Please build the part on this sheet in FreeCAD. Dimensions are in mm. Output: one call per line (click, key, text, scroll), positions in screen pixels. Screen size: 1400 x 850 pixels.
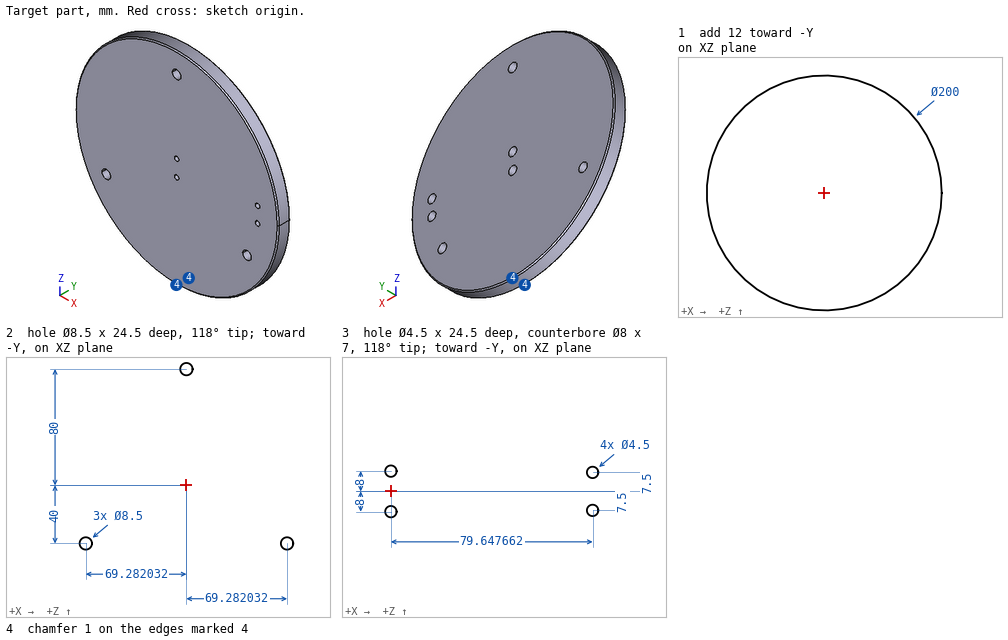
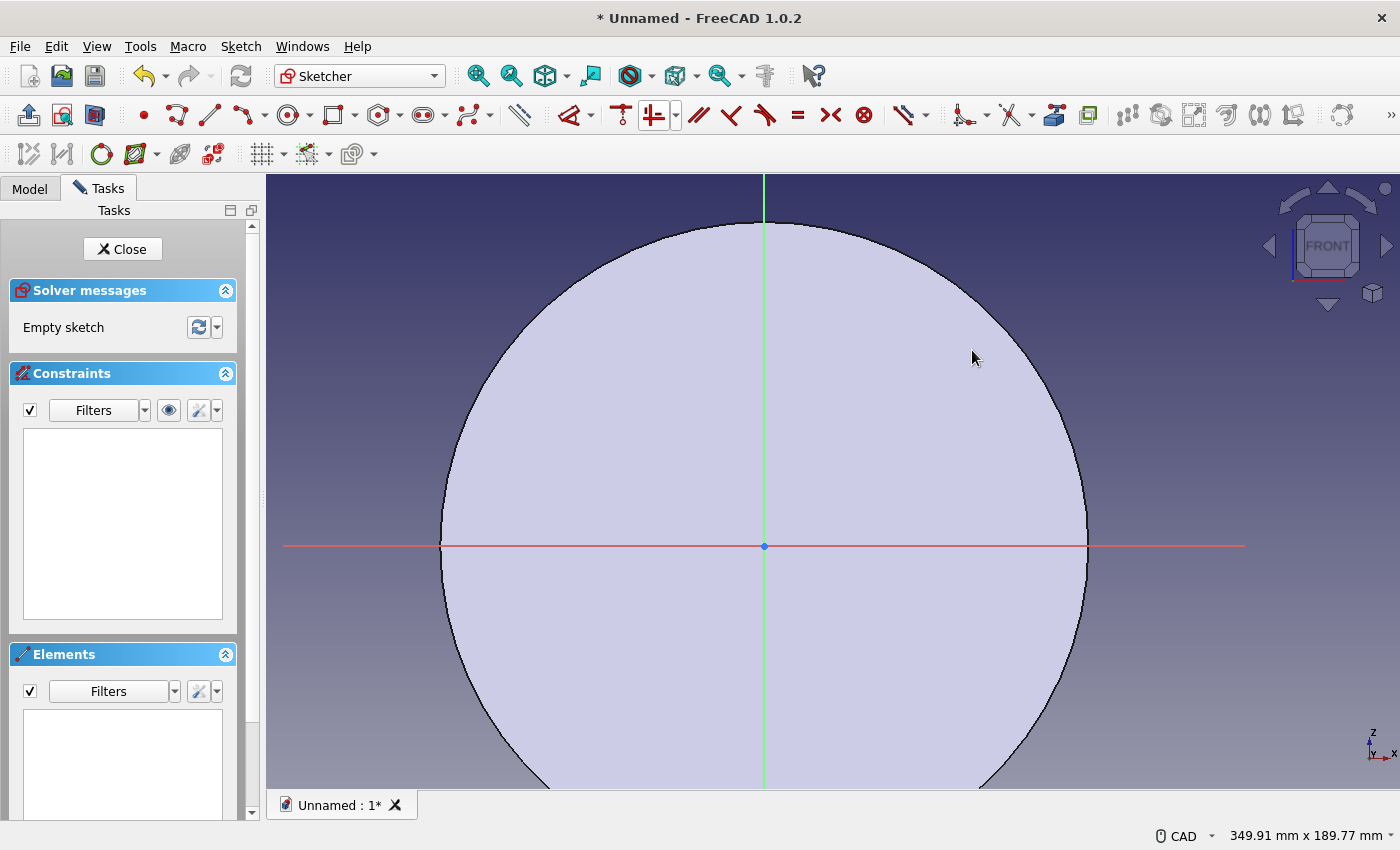
click(288, 116)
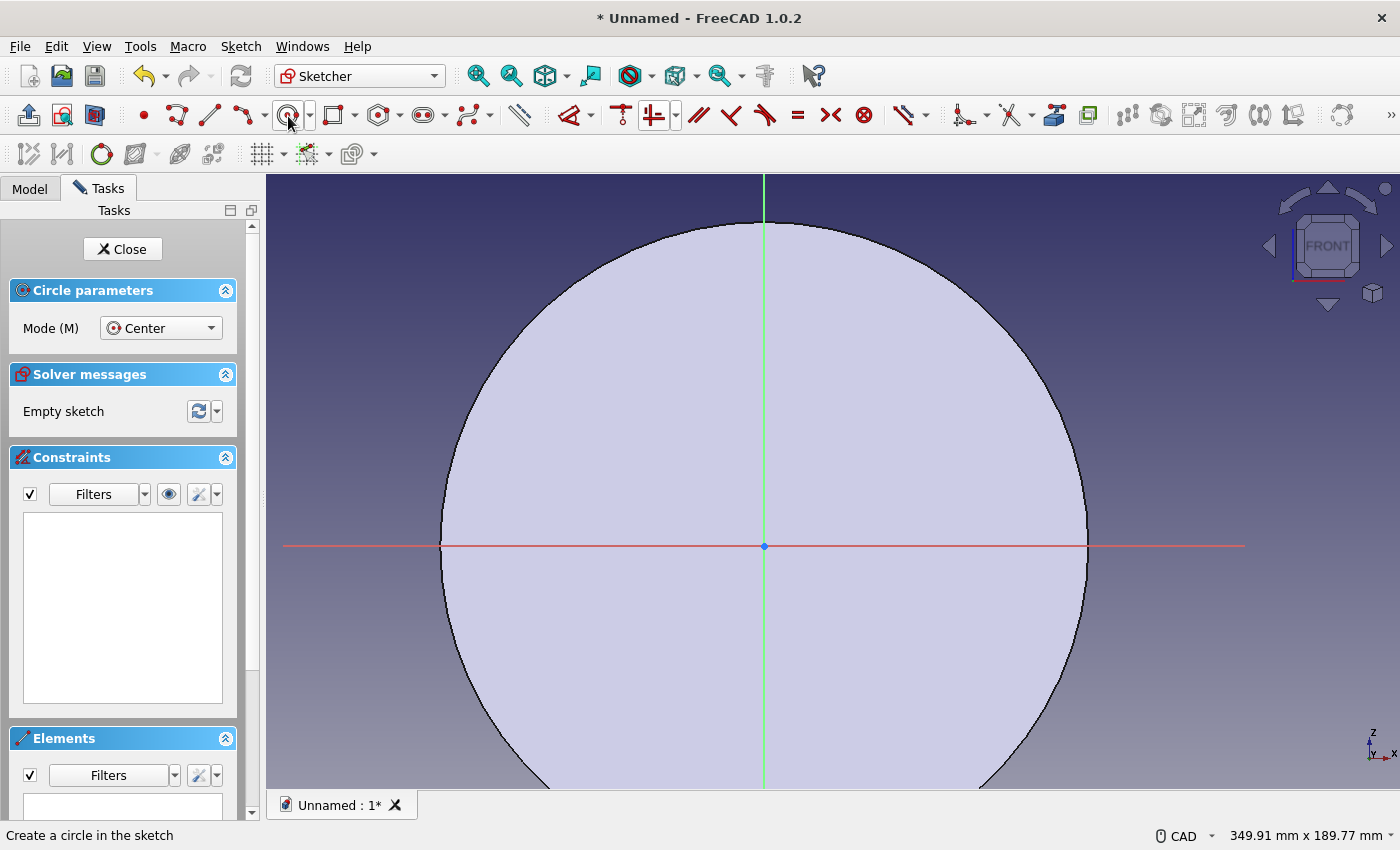
scroll(540, 676, up, 3)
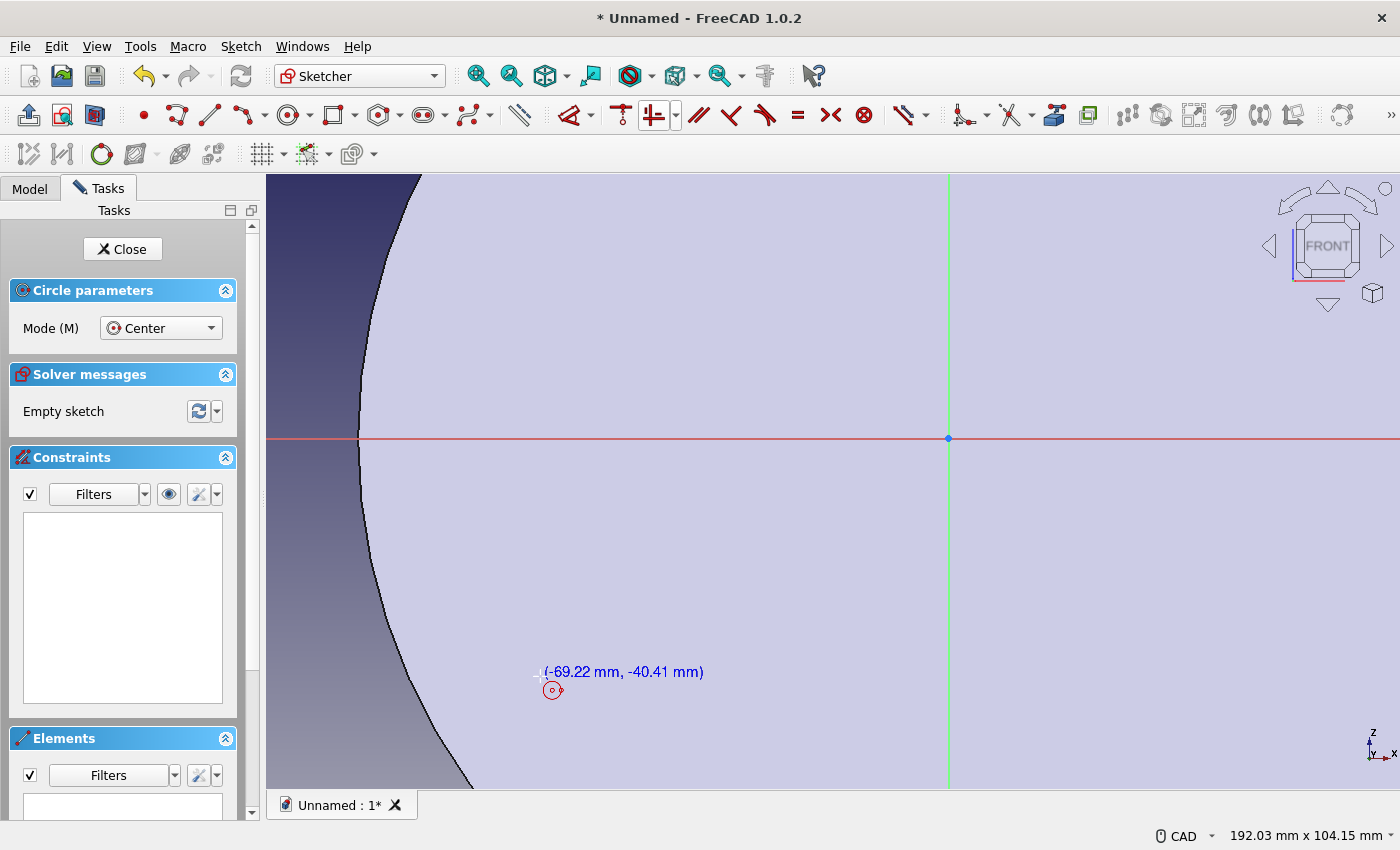
click(539, 675)
move(557, 657)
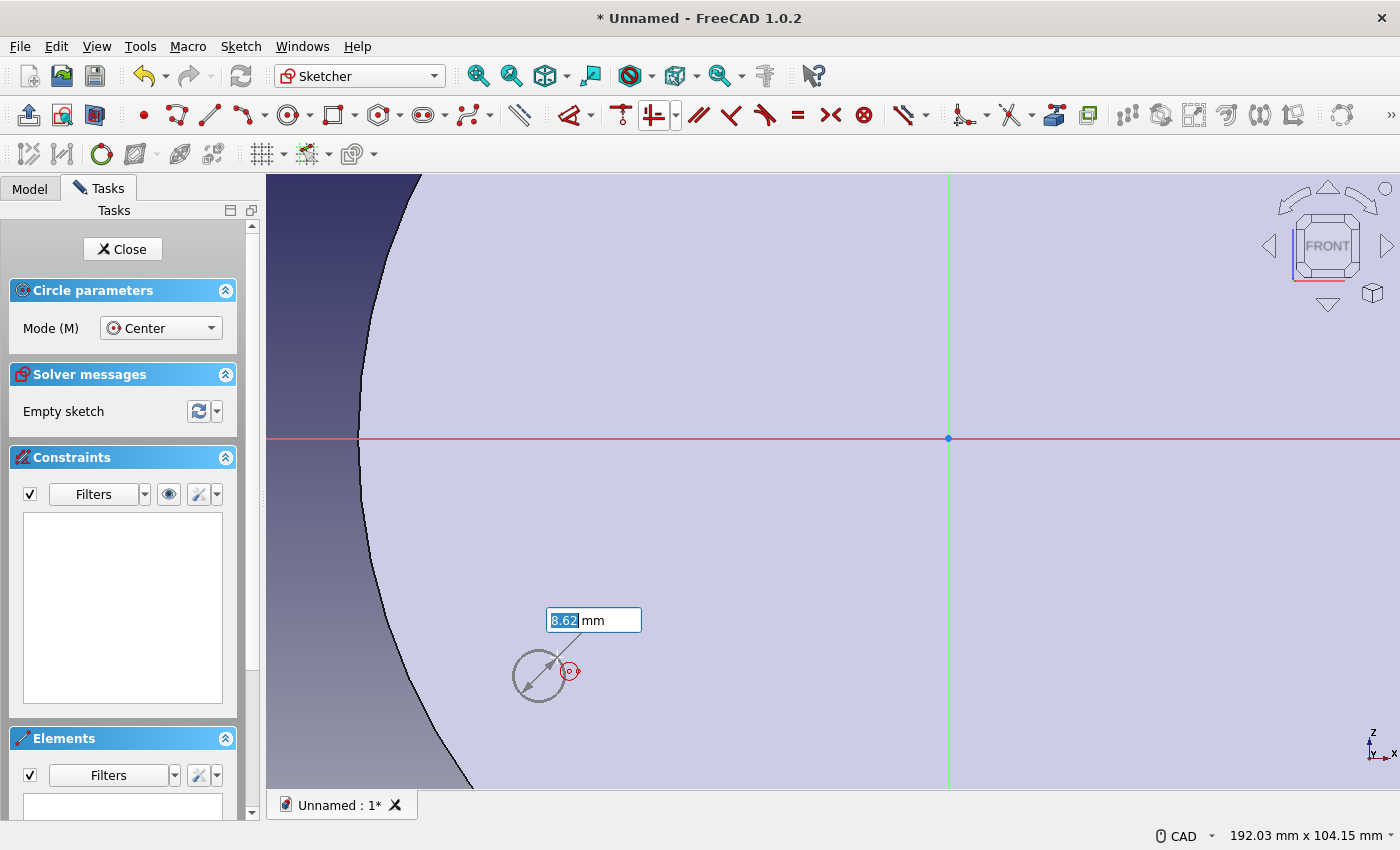
text(8.5)
key(Return)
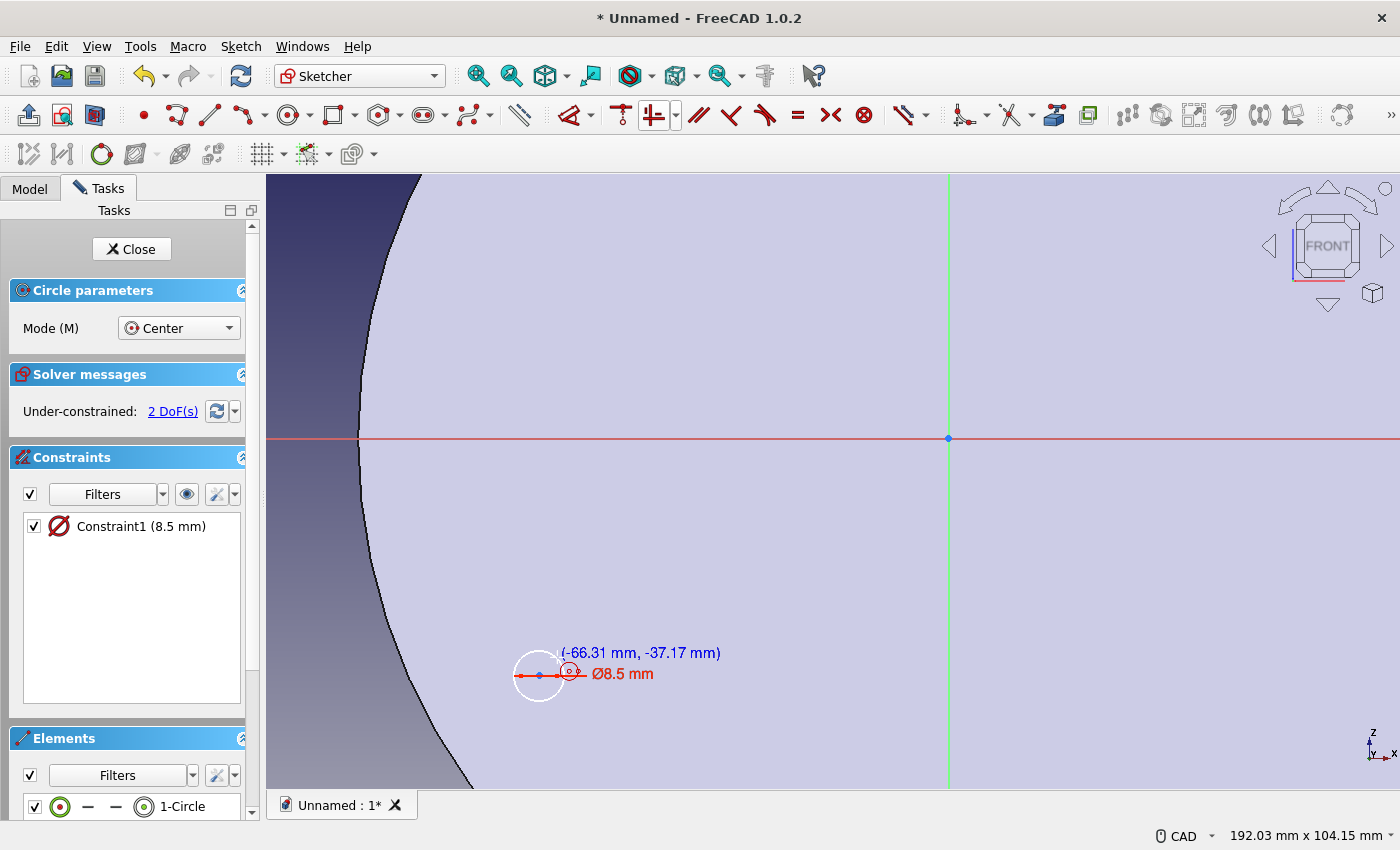
scroll(541, 677, down, 3)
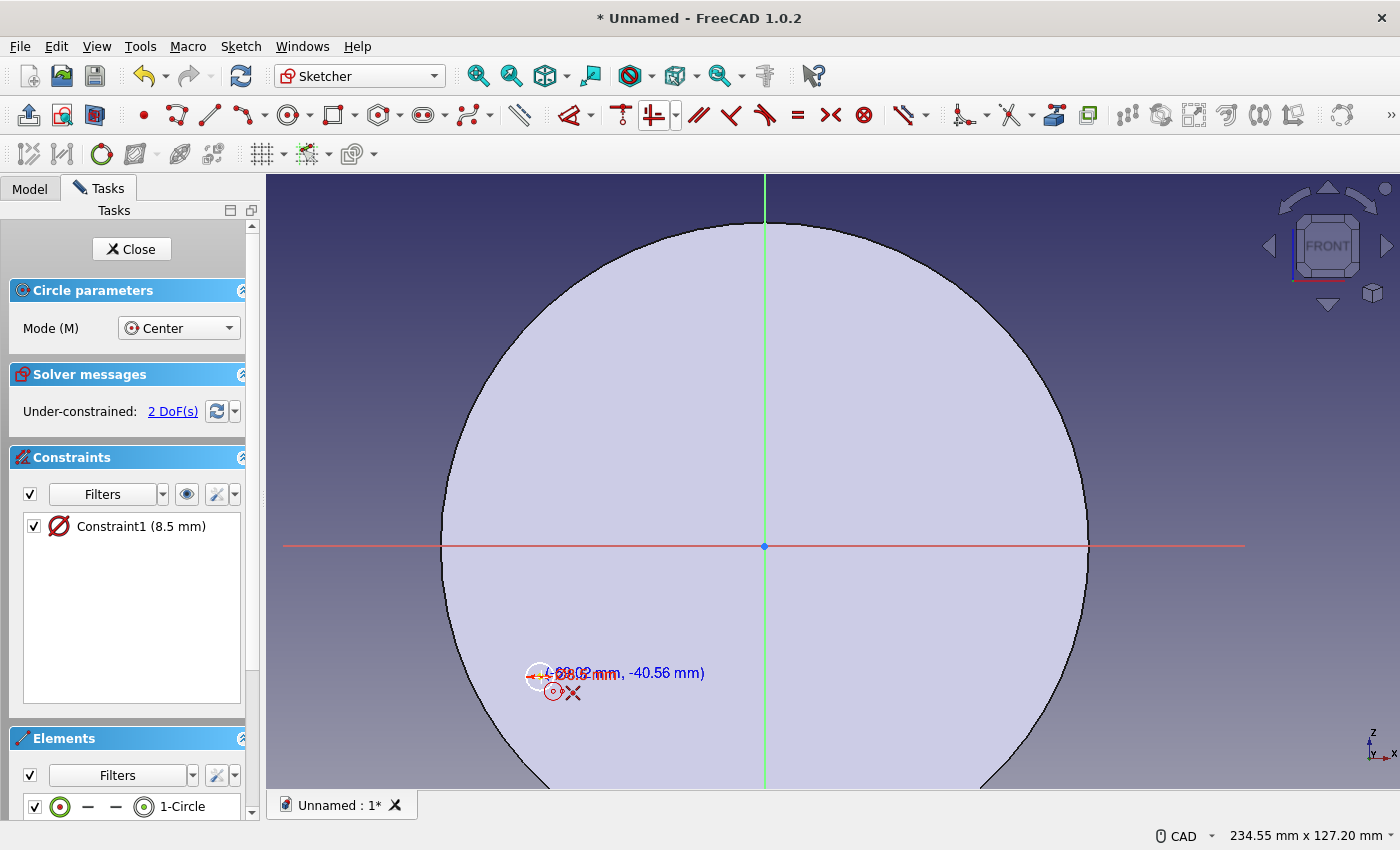
scroll(989, 676, up, 3)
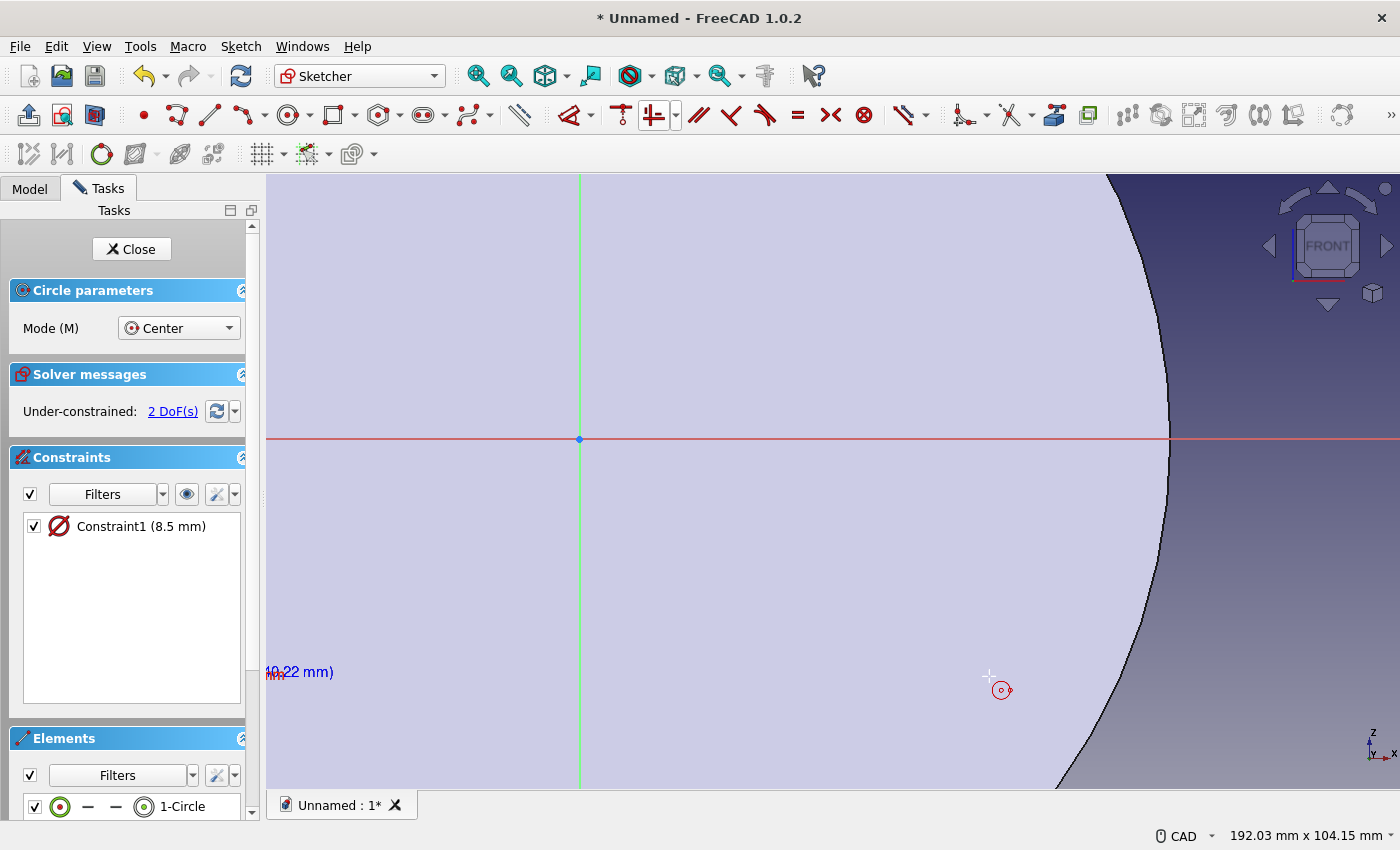
click(989, 676)
move(1007, 658)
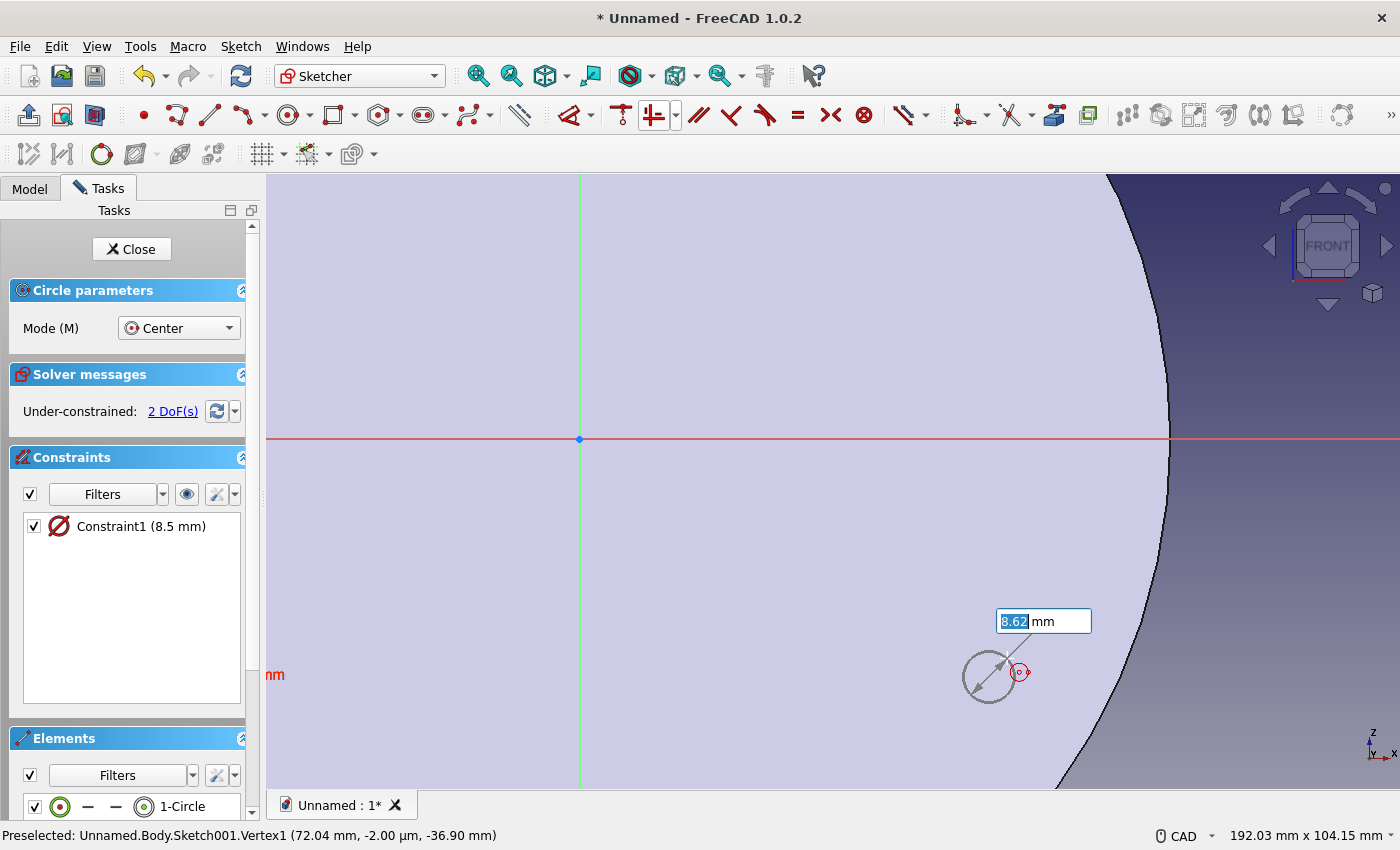
text(8.5)
key(Return)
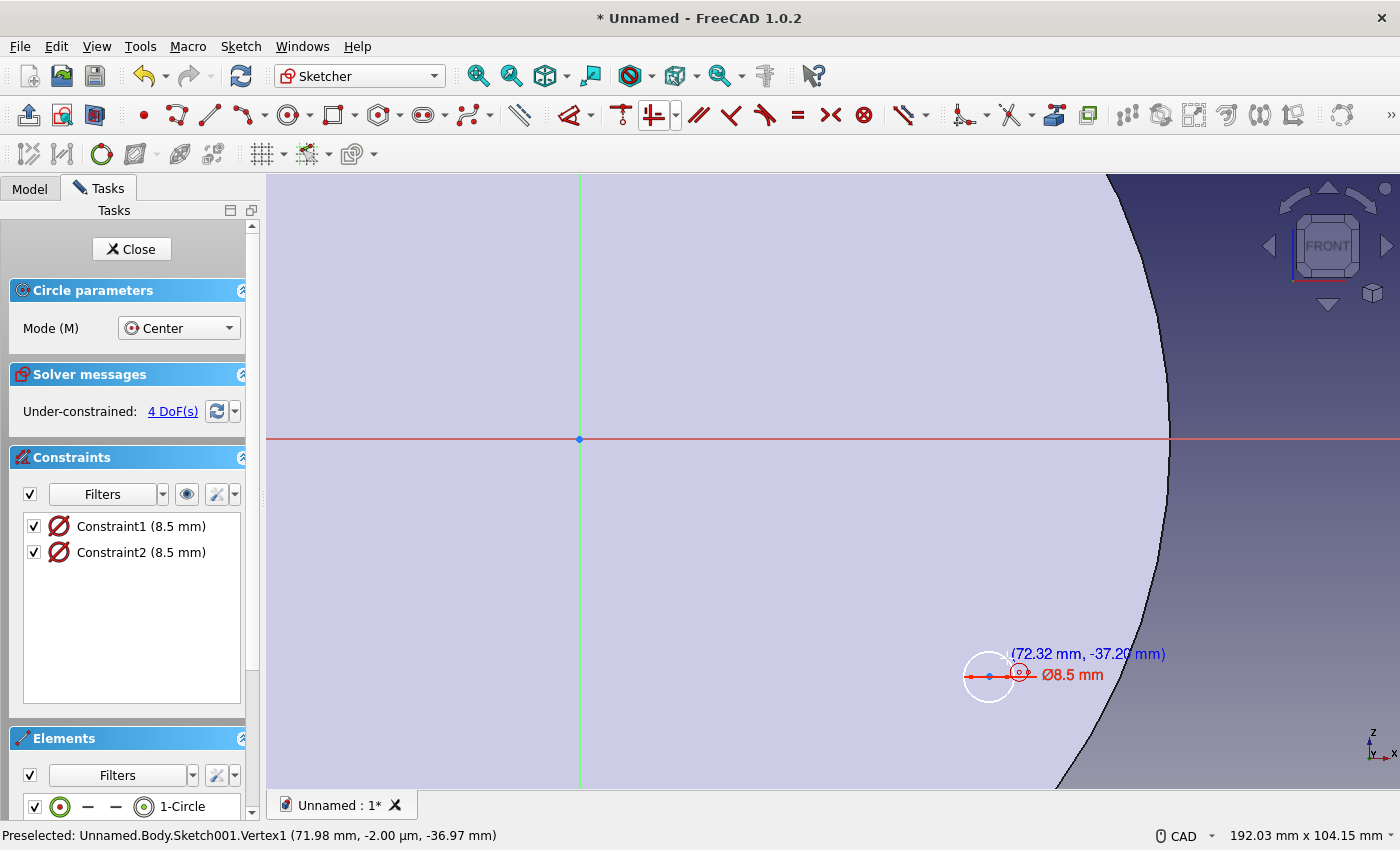
scroll(989, 676, down, 3)